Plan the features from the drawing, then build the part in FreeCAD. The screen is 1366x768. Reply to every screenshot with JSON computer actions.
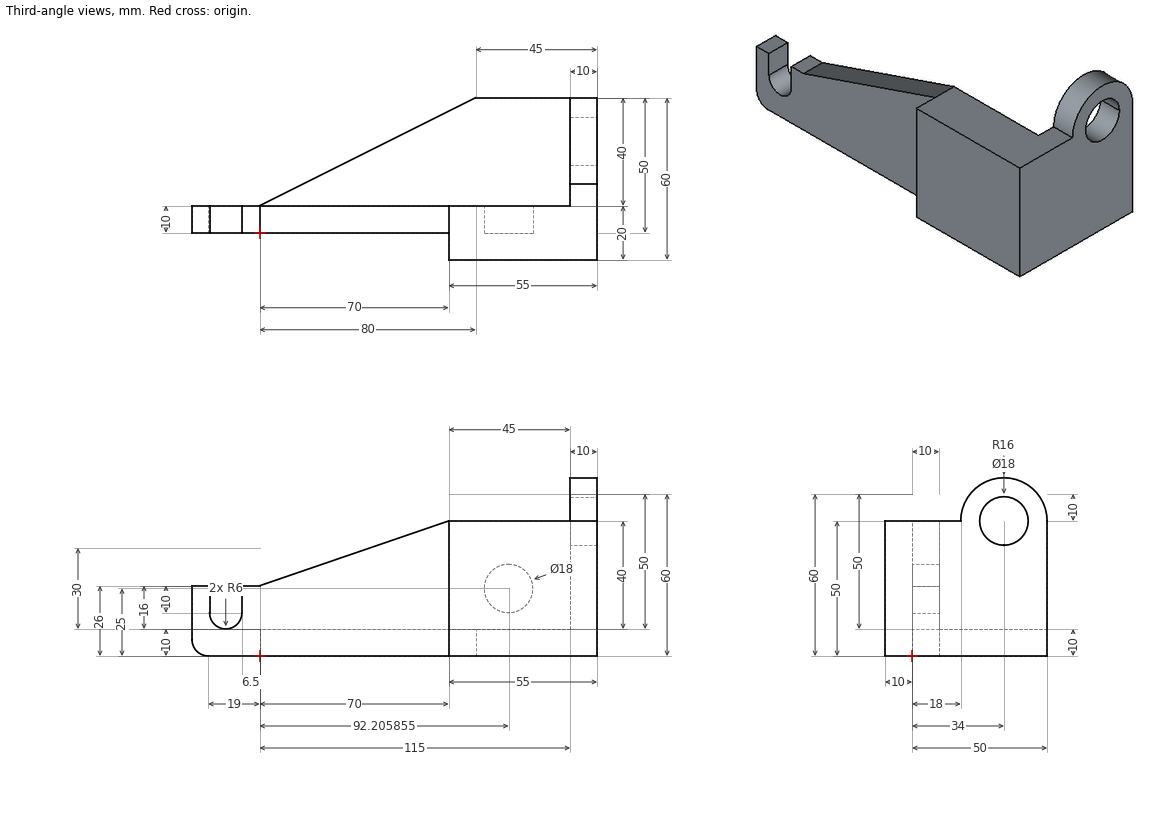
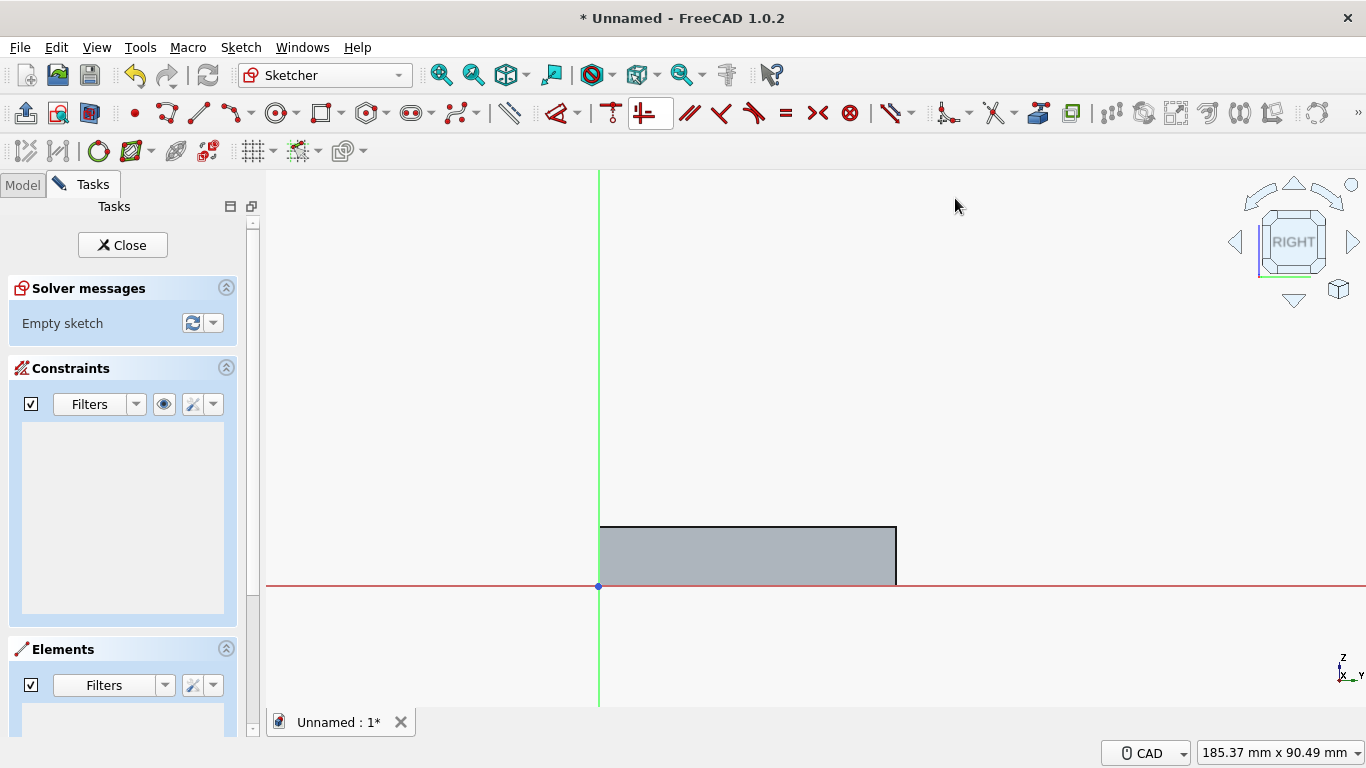
{"action": "left_click", "coordinate": [322, 114]}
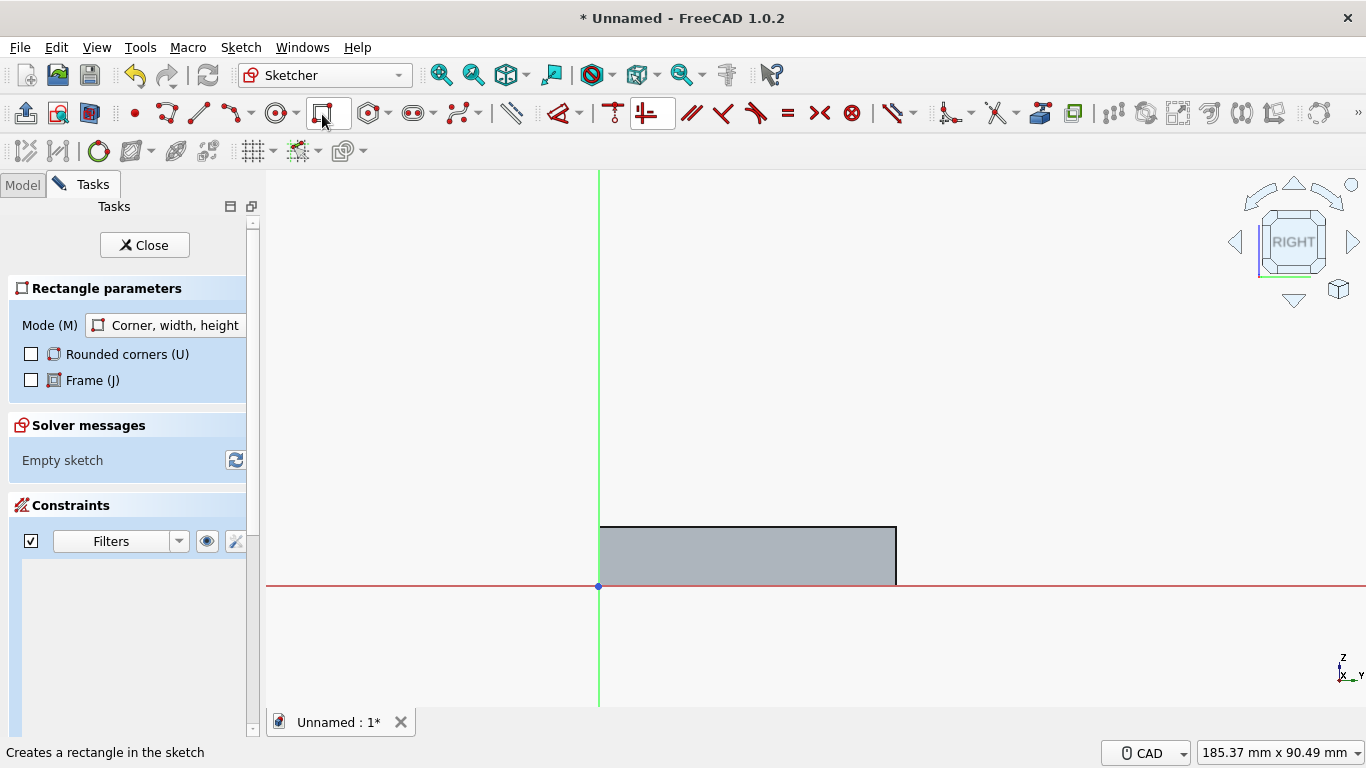
{"action": "left_click", "coordinate": [599, 230]}
{"action": "left_click", "coordinate": [896, 527]}
{"action": "key", "text": "Escape"}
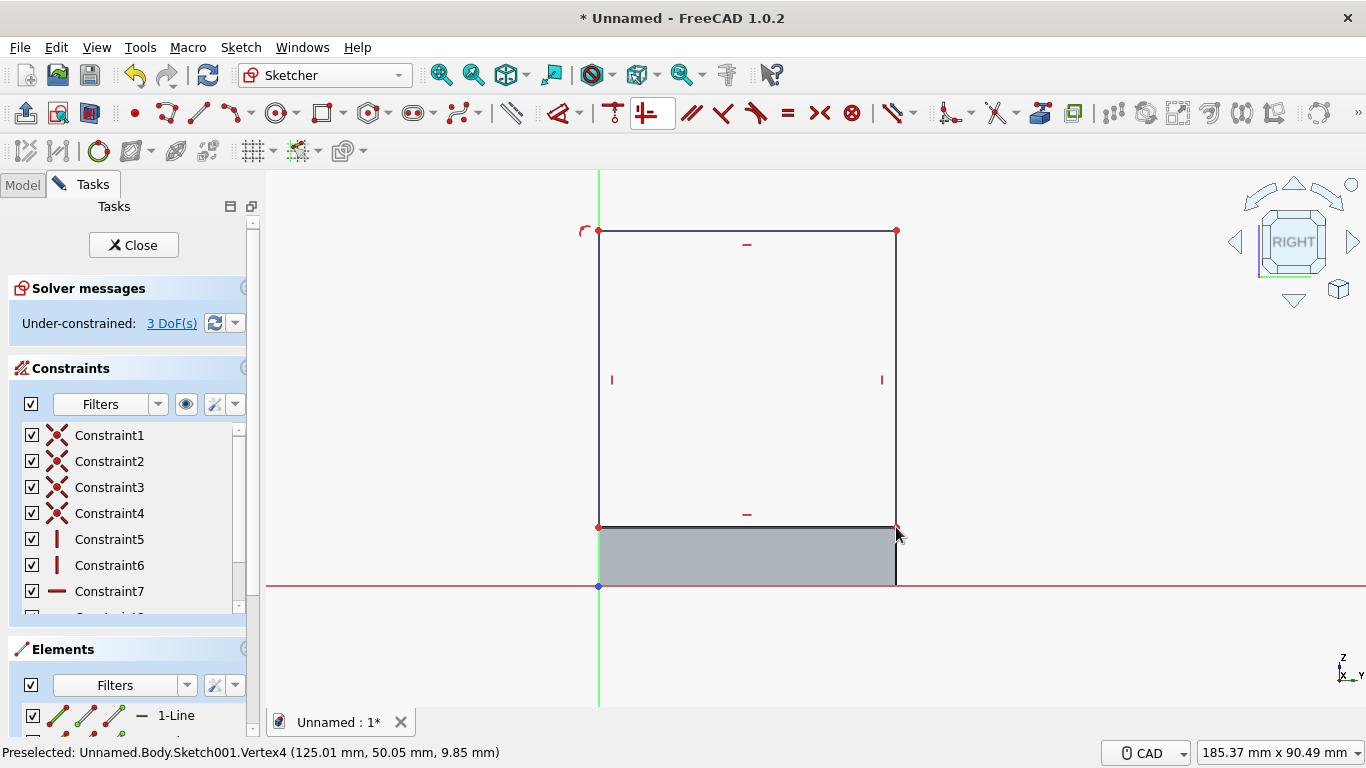
{"action": "left_click", "coordinate": [558, 114]}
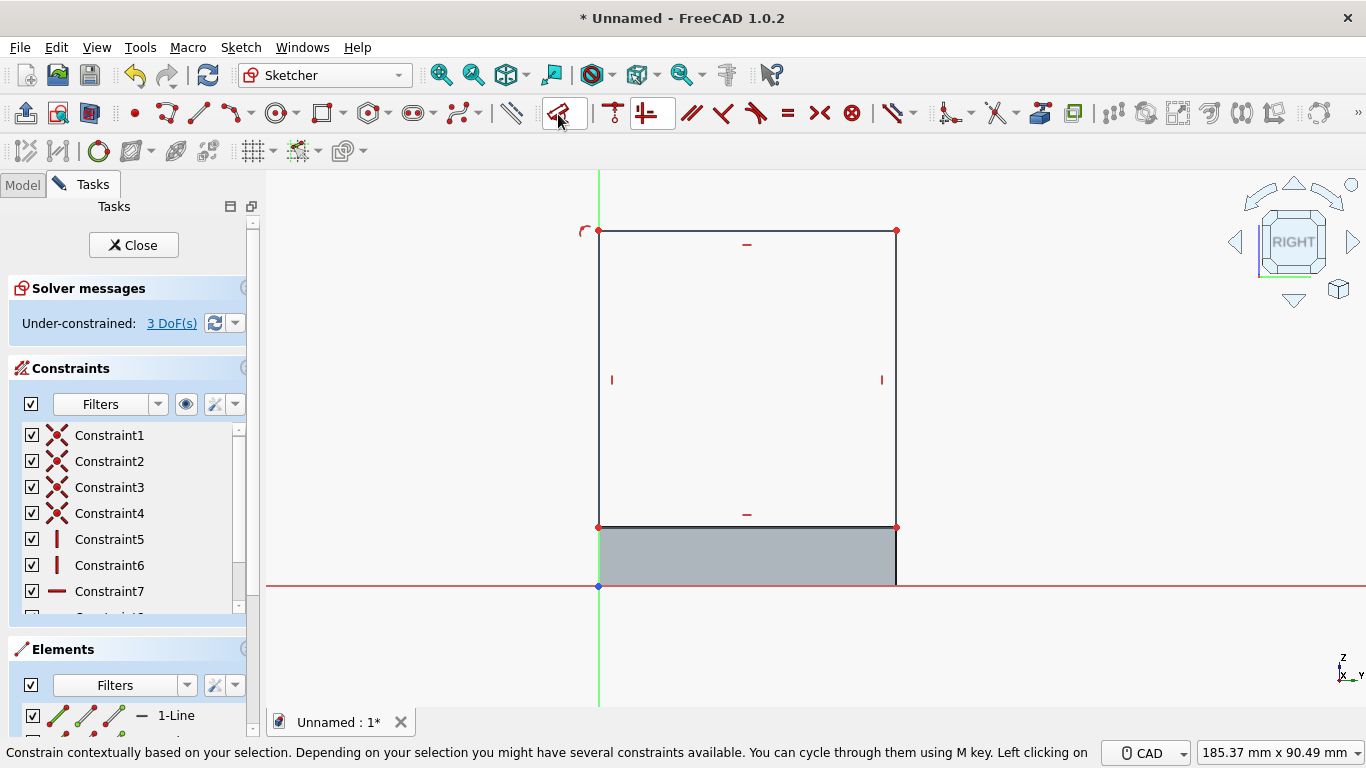
{"action": "left_click", "coordinate": [599, 320]}
{"action": "left_click", "coordinate": [565, 380]}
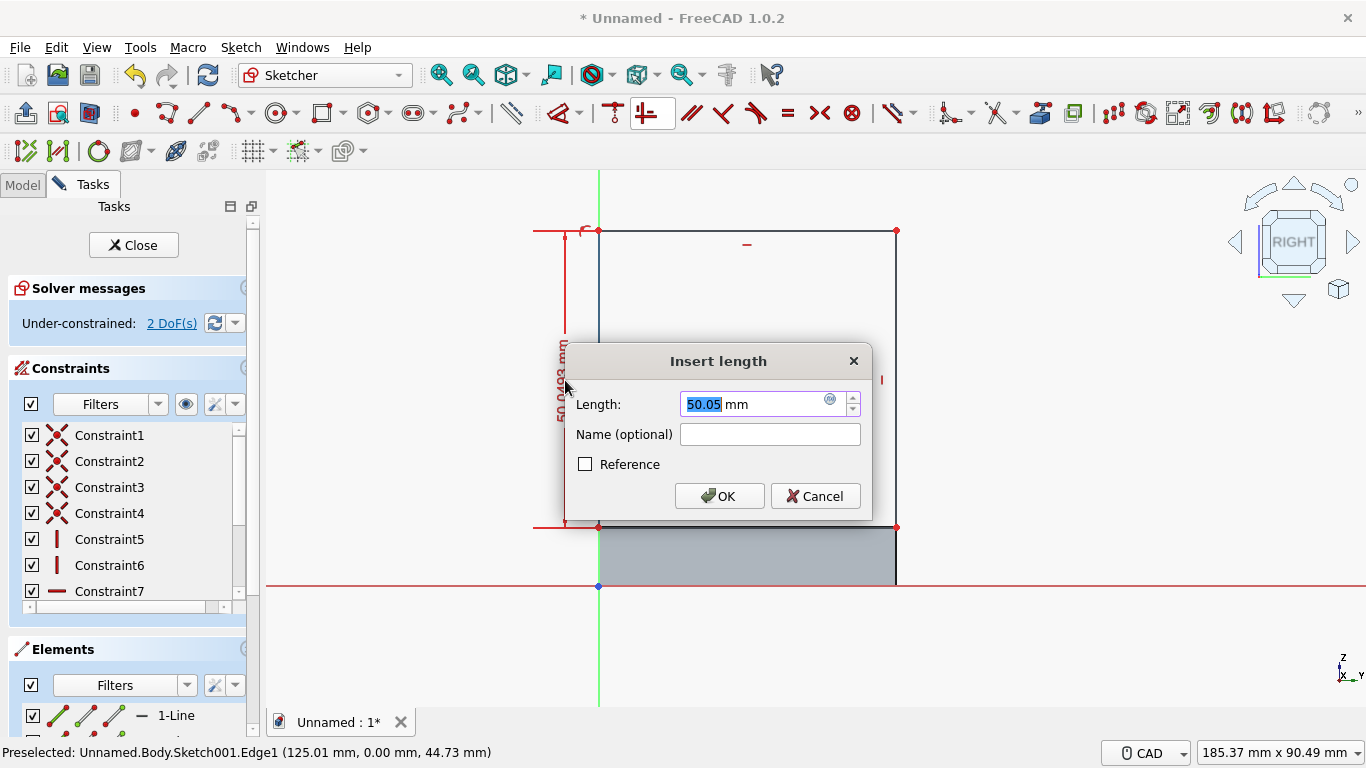
{"action": "type", "text": "50"}
{"action": "key", "text": "Return"}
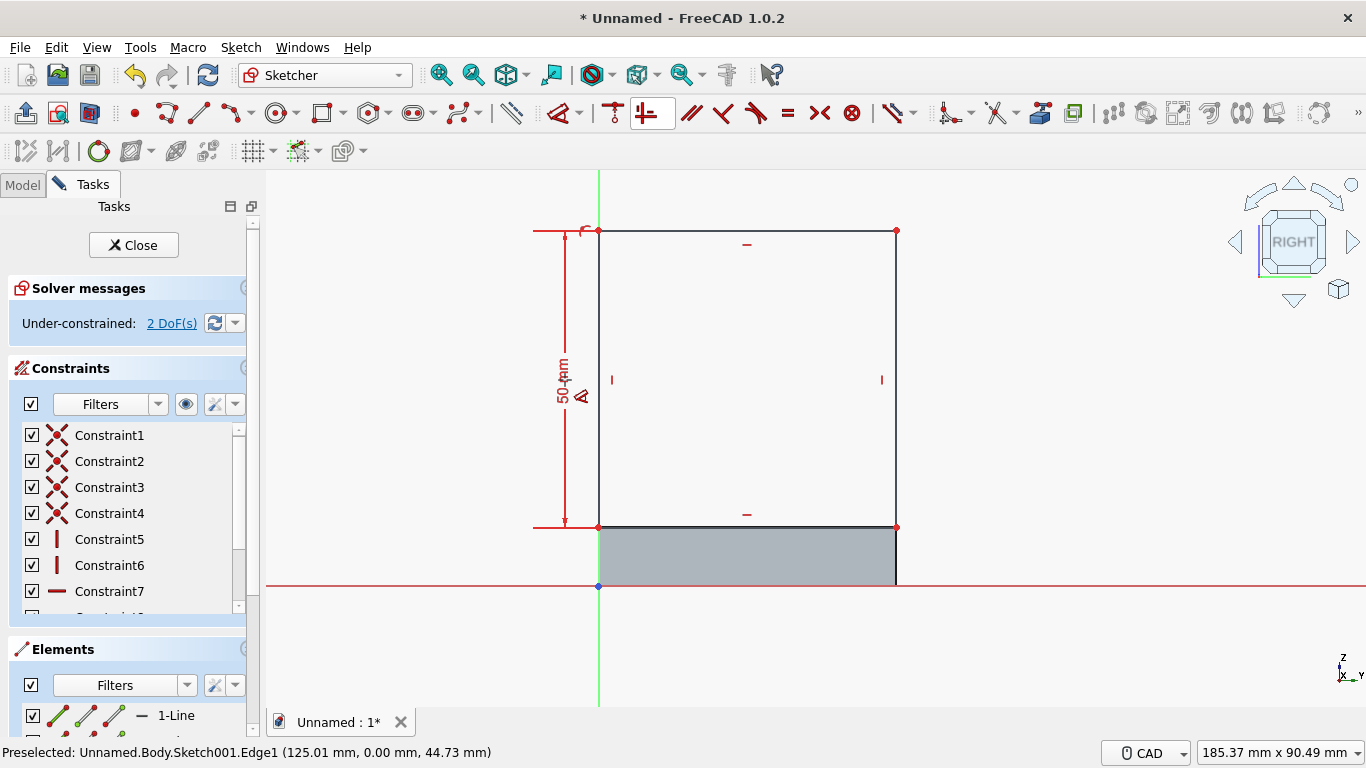
{"action": "left_click", "coordinate": [688, 528]}
{"action": "left_click", "coordinate": [747, 562]}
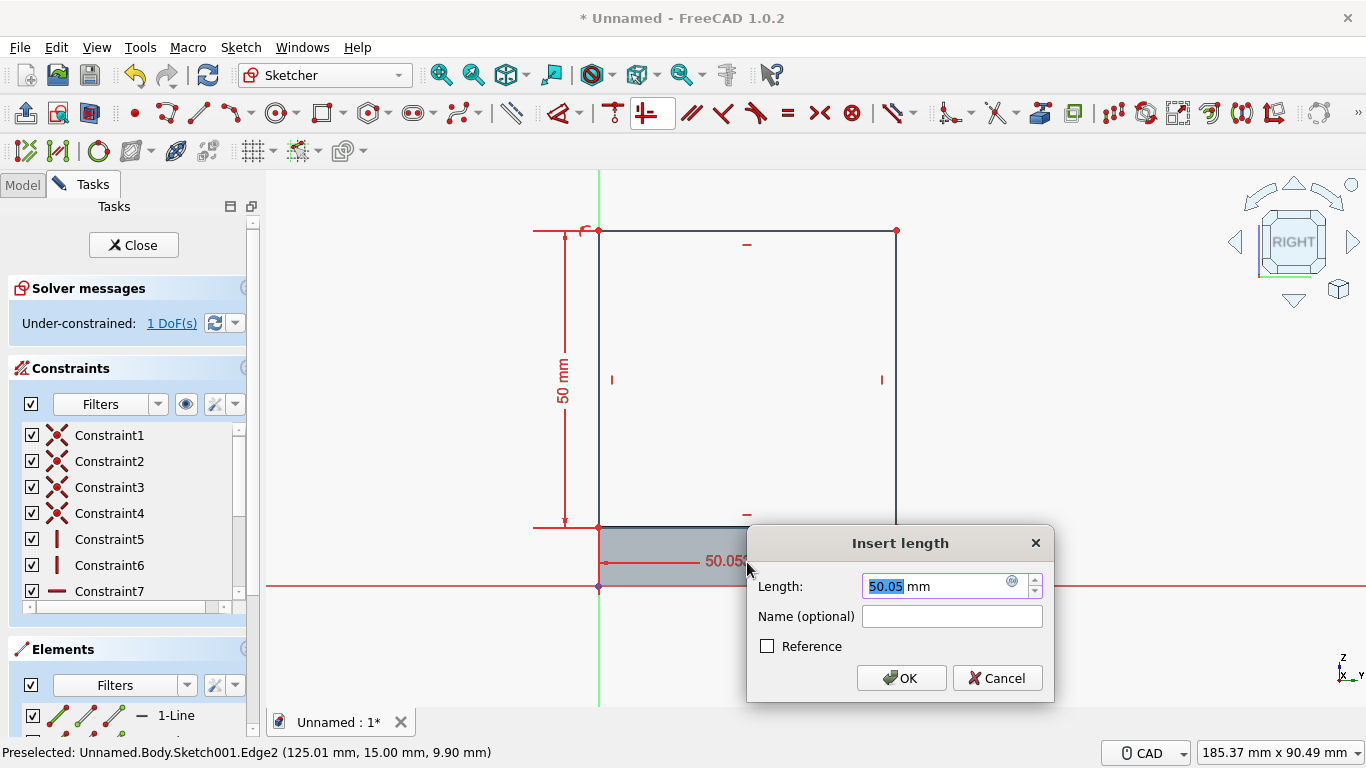
{"action": "type", "text": "50"}
{"action": "key", "text": "Return"}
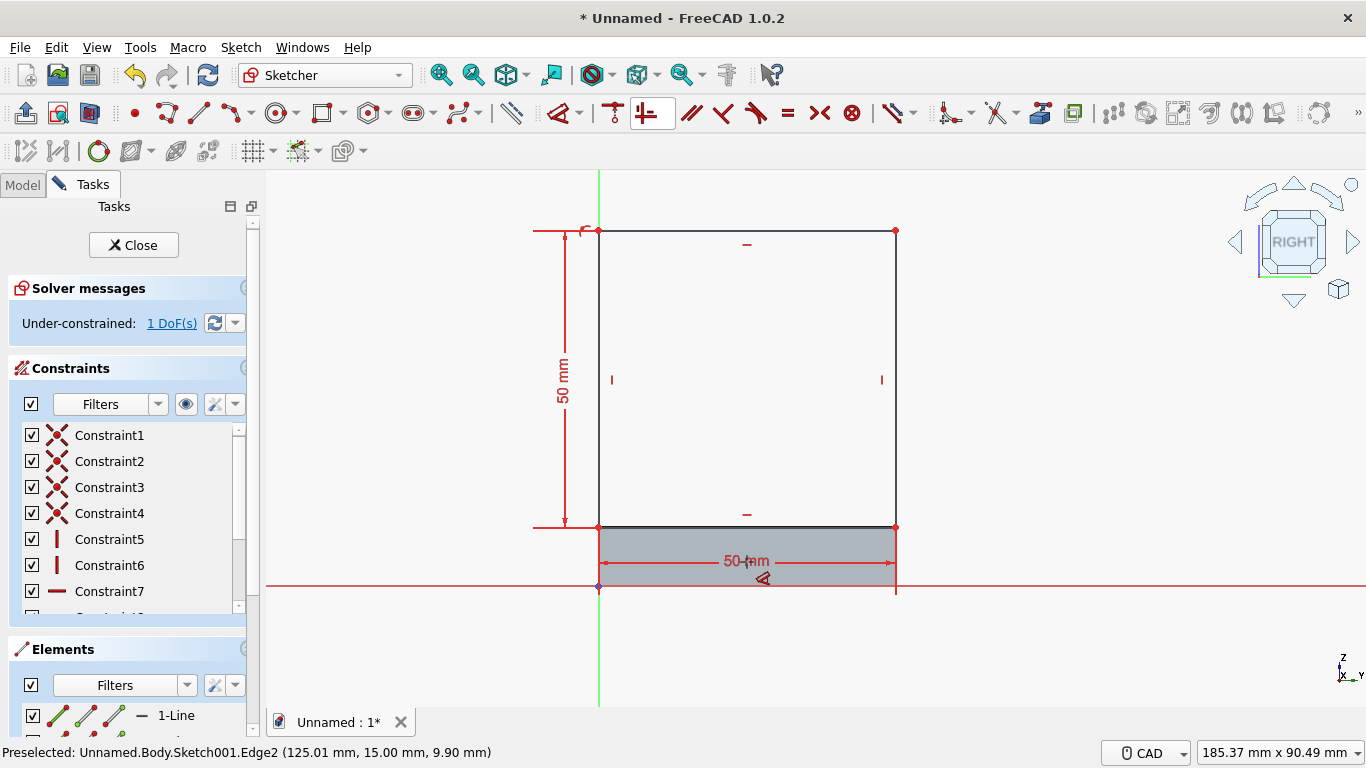
{"action": "left_click", "coordinate": [599, 231]}
{"action": "left_click", "coordinate": [565, 409]}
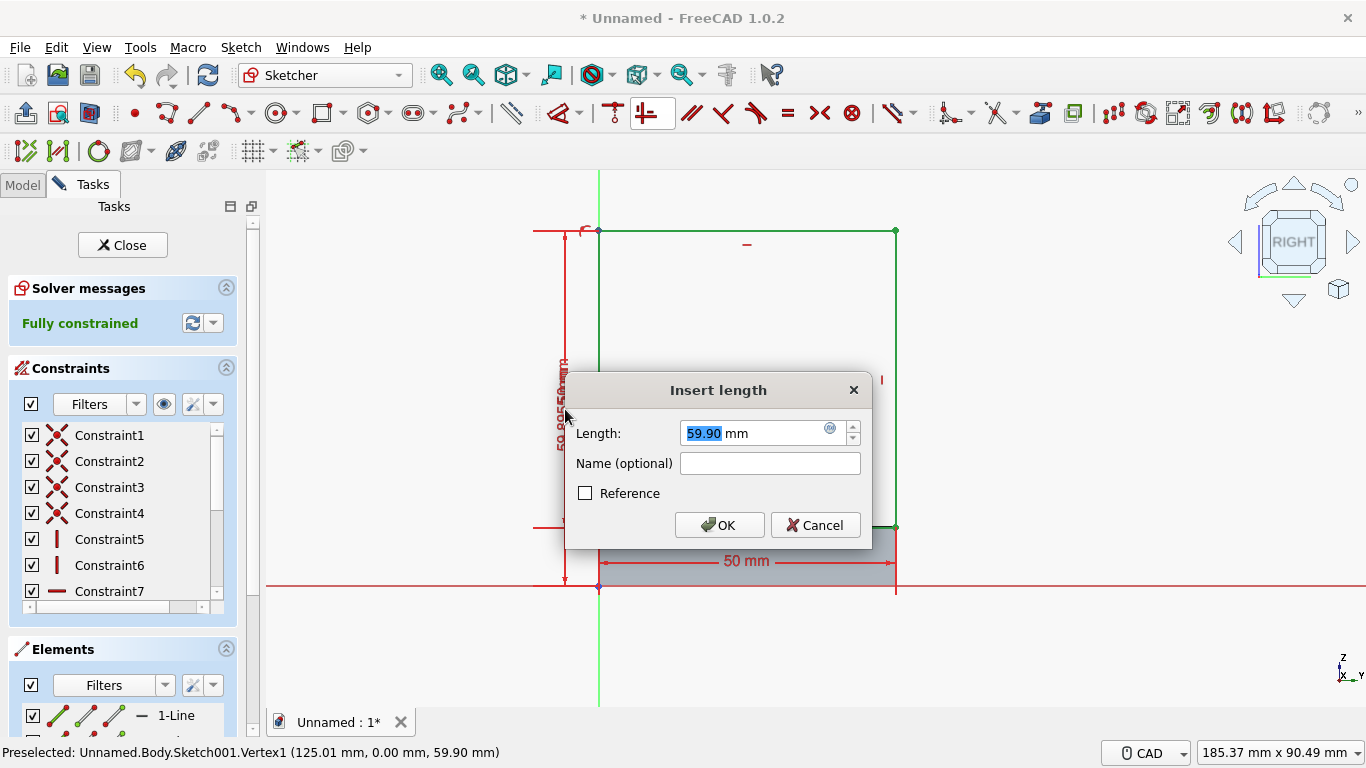
{"action": "type", "text": "60"}
{"action": "key", "text": "Return"}
{"action": "key", "text": "Escape"}